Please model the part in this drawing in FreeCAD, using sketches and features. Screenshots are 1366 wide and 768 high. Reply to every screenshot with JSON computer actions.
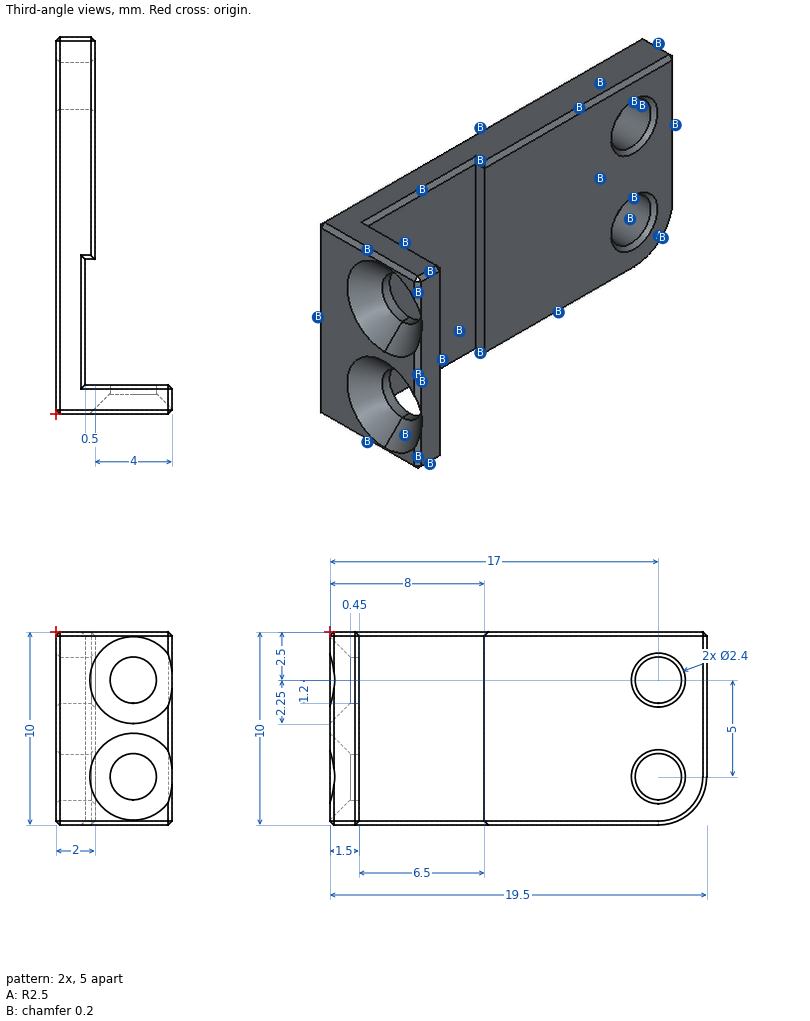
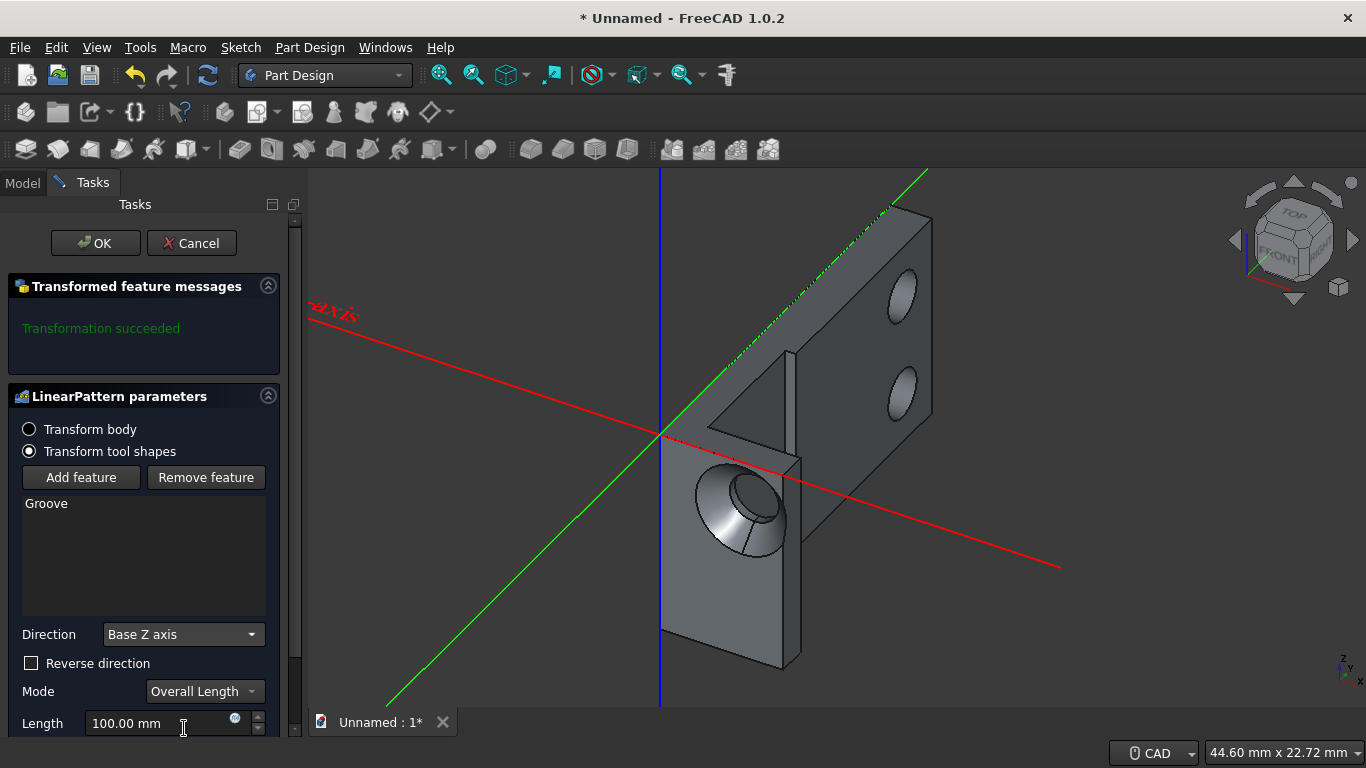
{"action": "left_click", "coordinate": [206, 692]}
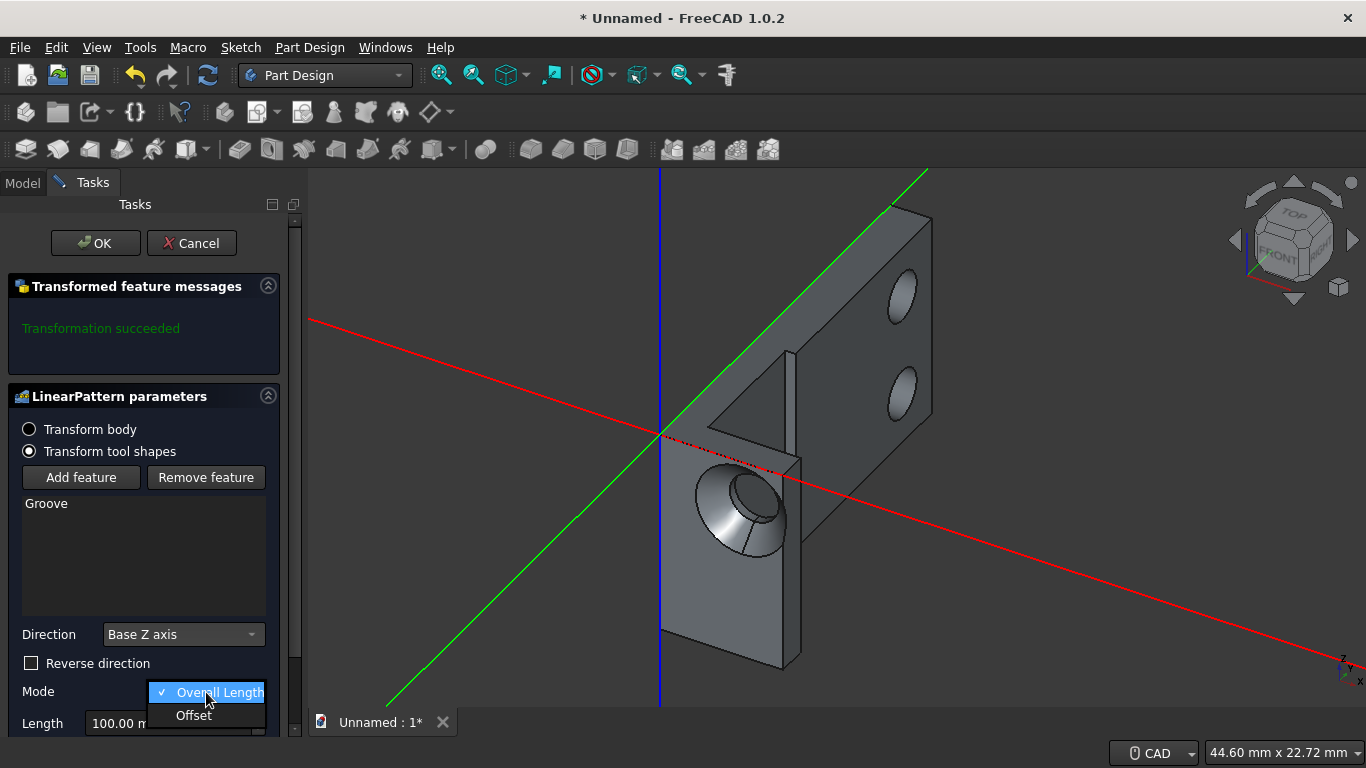
{"action": "left_click", "coordinate": [206, 716]}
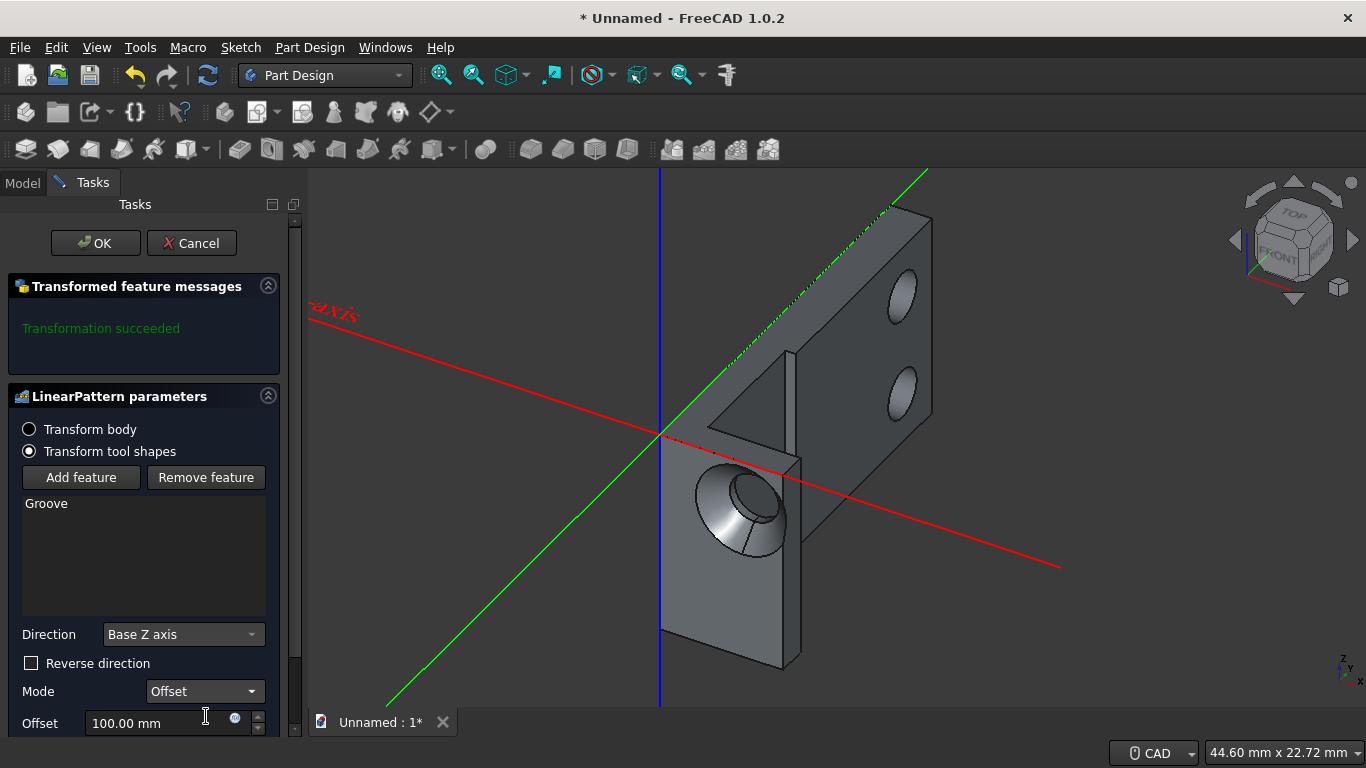
{"action": "triple_click", "coordinate": [168, 723]}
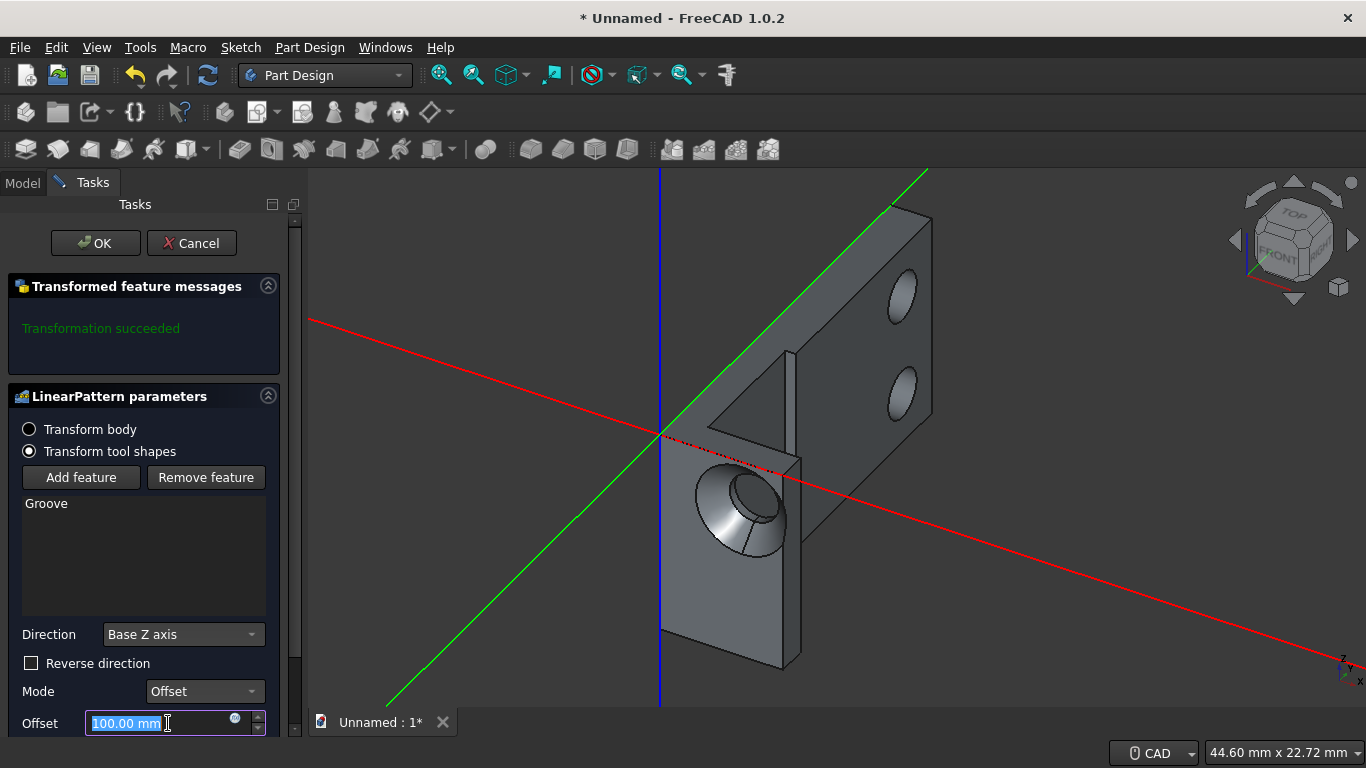
{"action": "type", "text": "5"}
{"action": "key", "text": "Tab"}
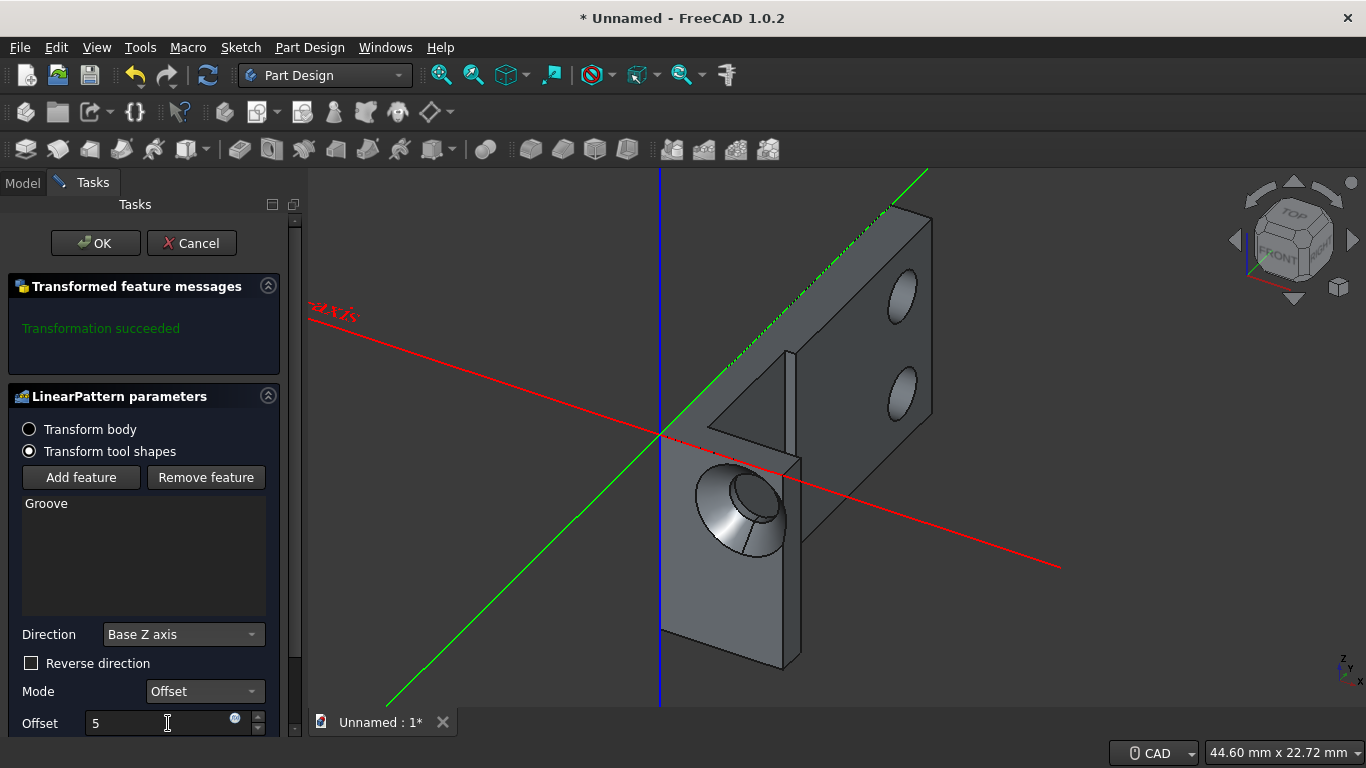
{"action": "scroll", "coordinate": [295, 475], "scroll_direction": "down", "scroll_amount": 2}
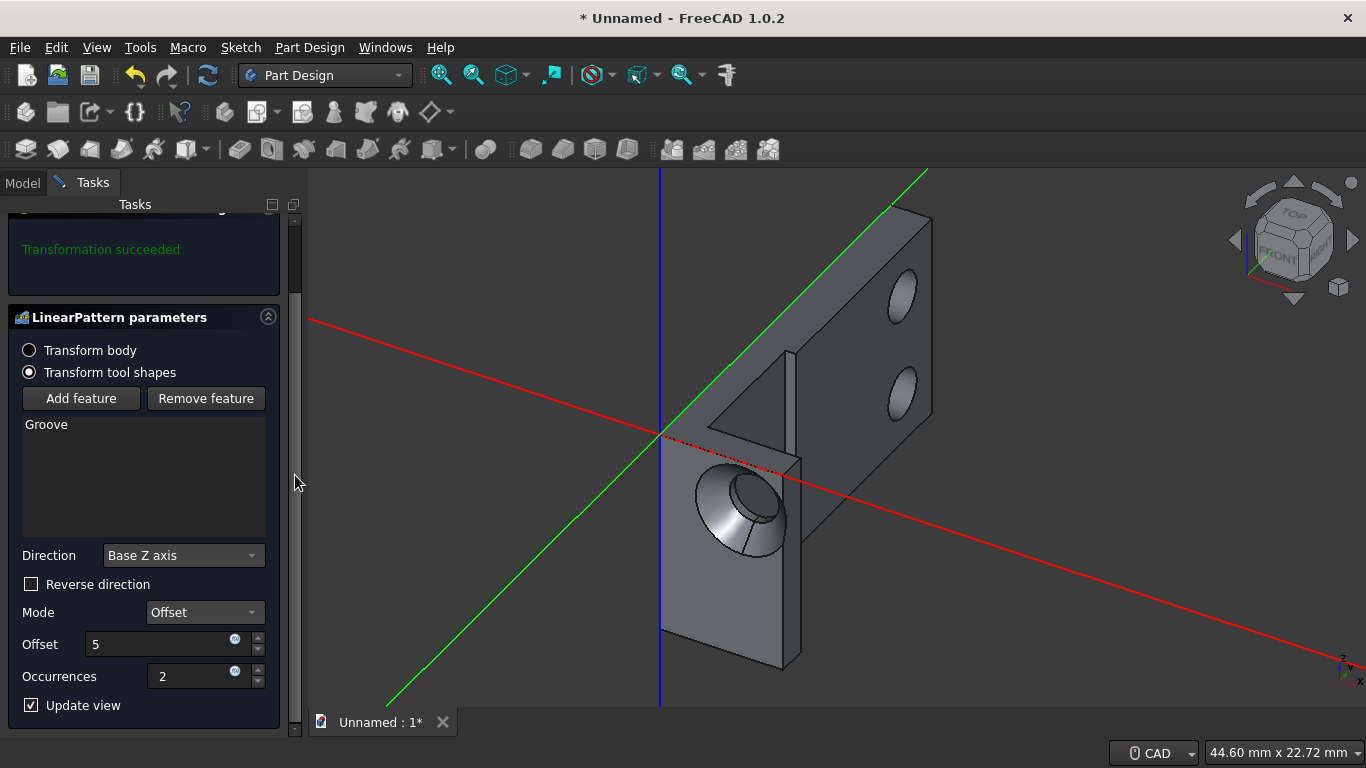
{"action": "triple_click", "coordinate": [198, 676]}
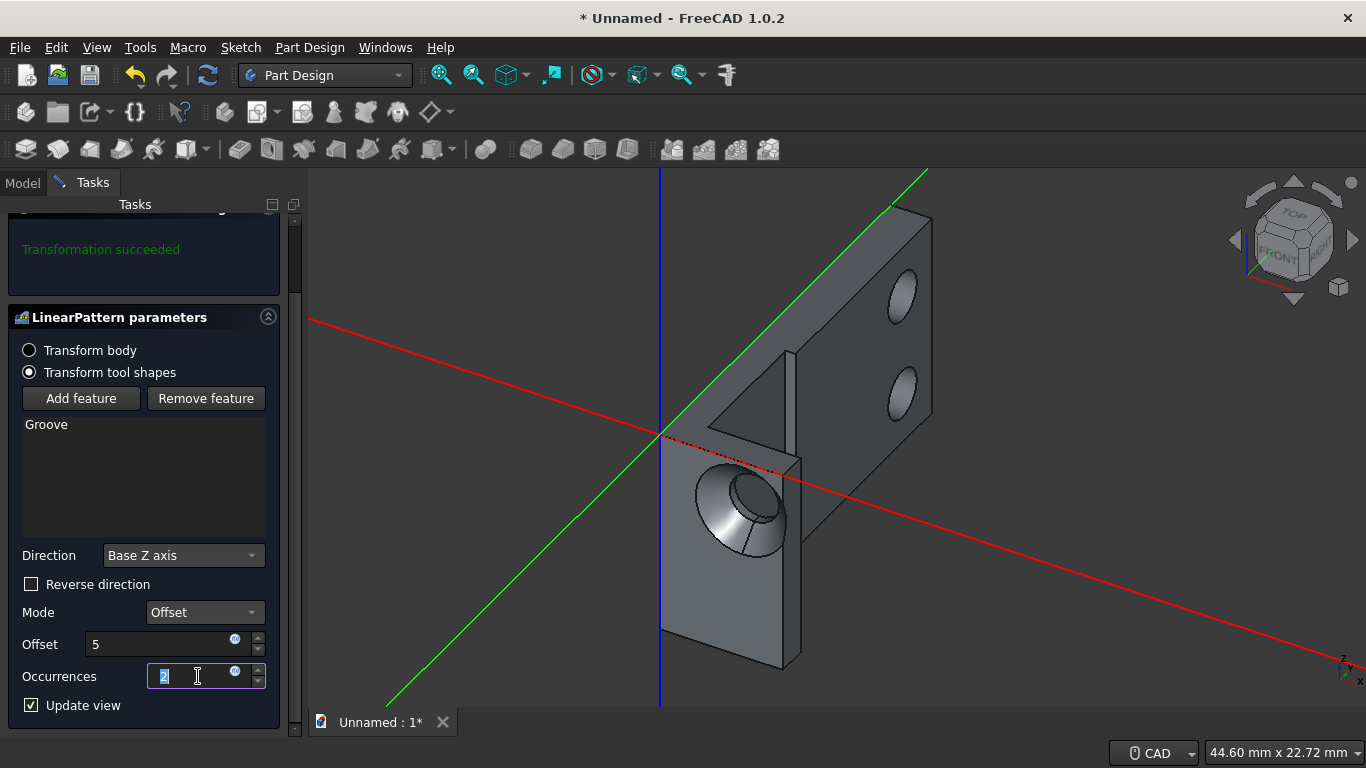
{"action": "type", "text": "2"}
{"action": "key", "text": "Tab"}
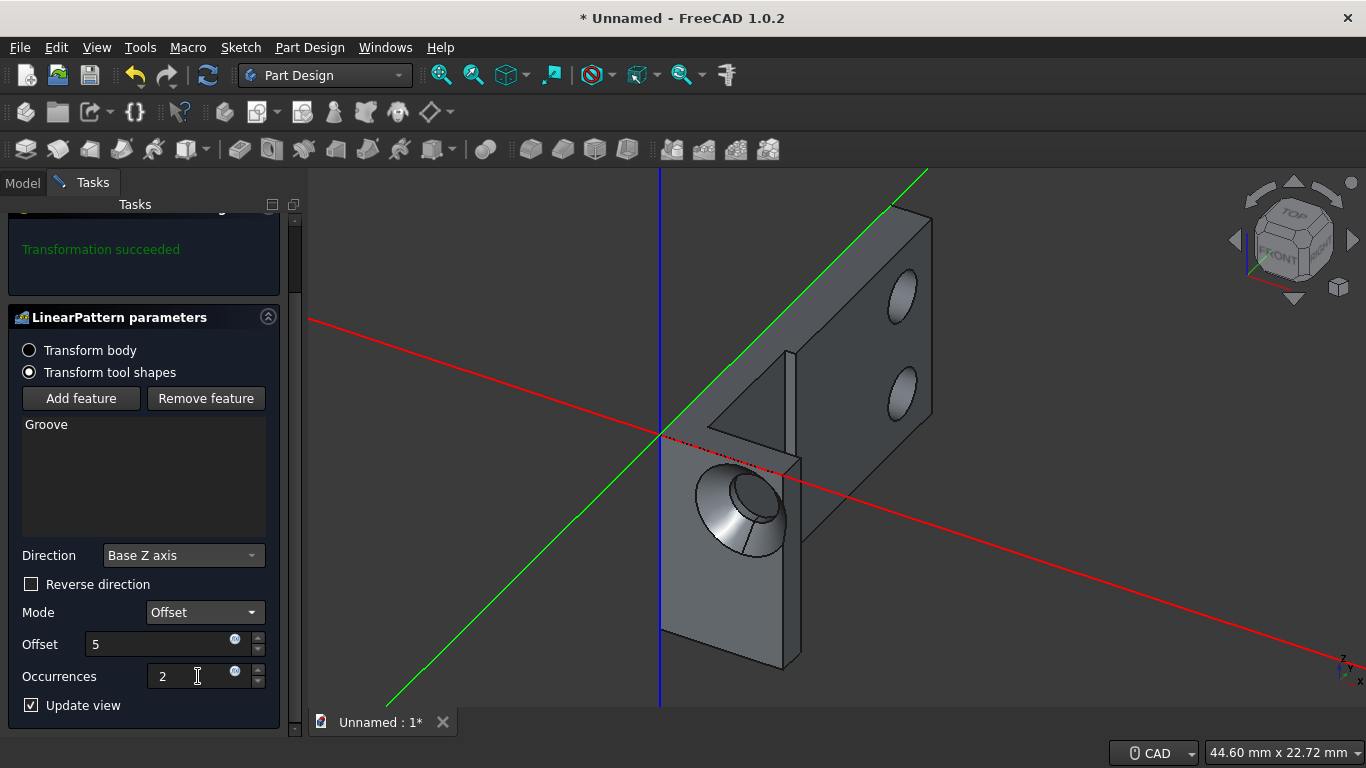
{"action": "left_click", "coordinate": [30, 584]}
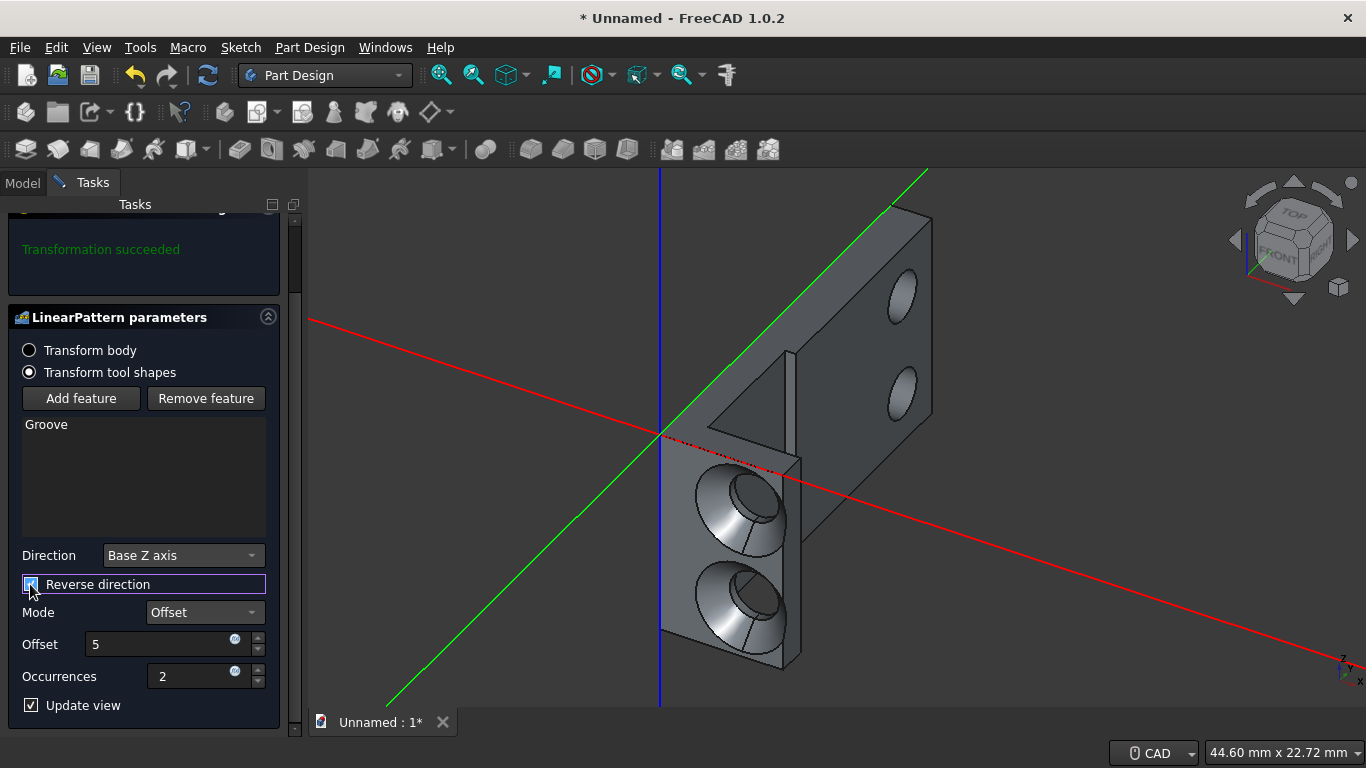
{"action": "scroll", "coordinate": [295, 475], "scroll_direction": "up", "scroll_amount": 3}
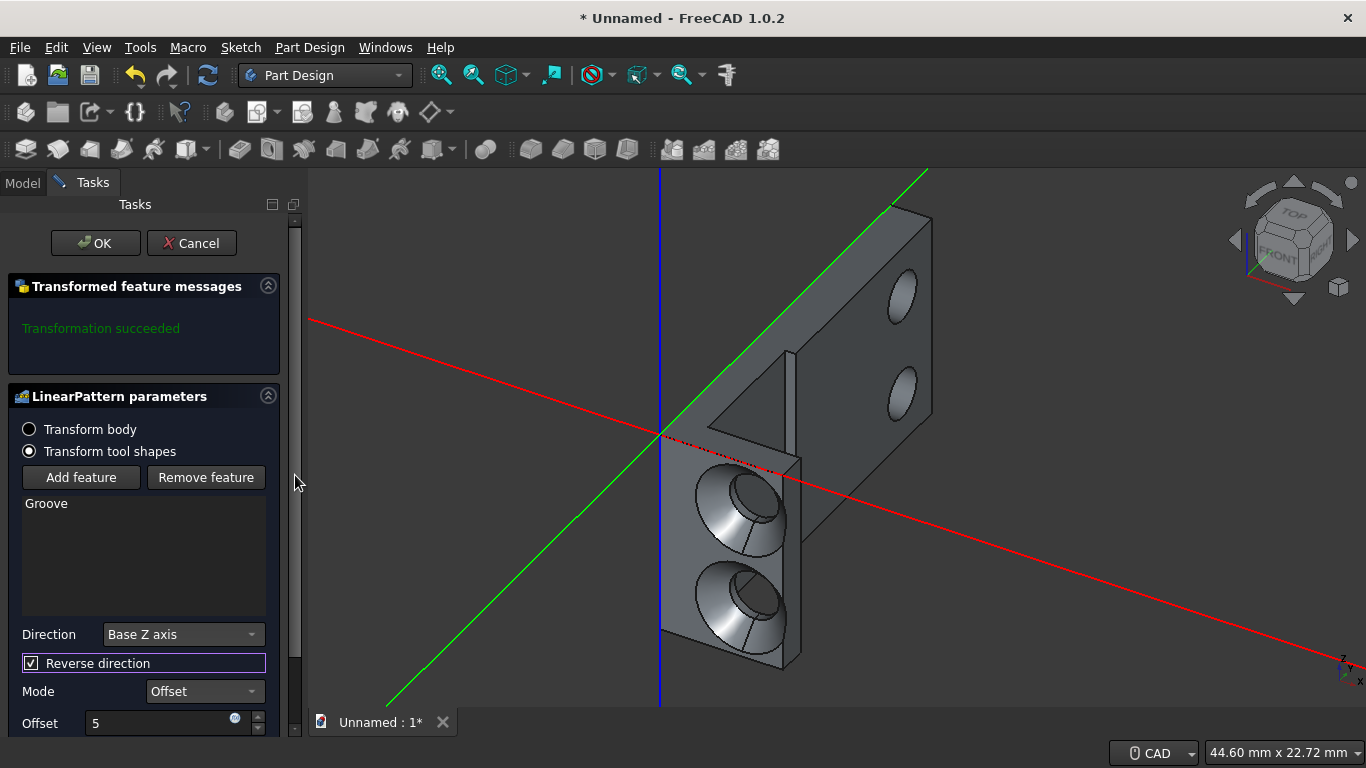
{"action": "left_click", "coordinate": [96, 243]}